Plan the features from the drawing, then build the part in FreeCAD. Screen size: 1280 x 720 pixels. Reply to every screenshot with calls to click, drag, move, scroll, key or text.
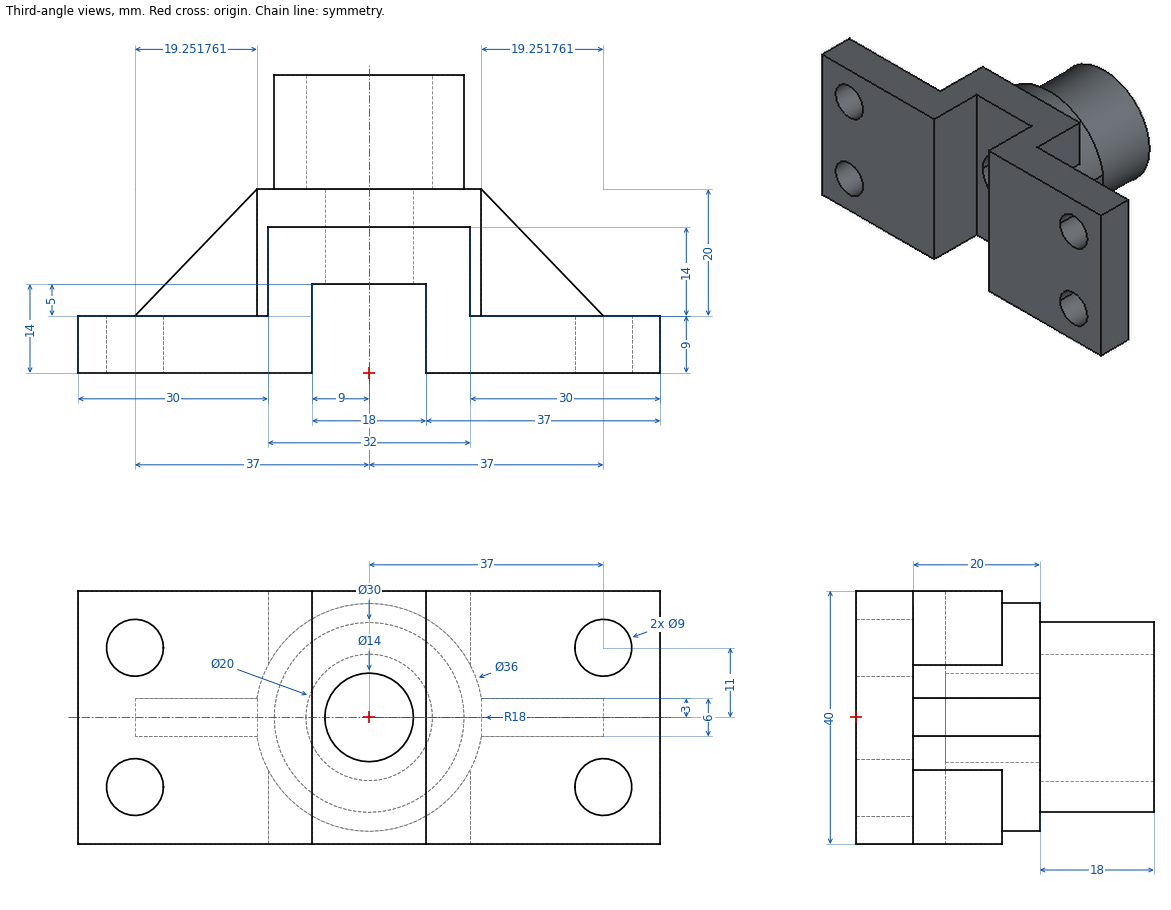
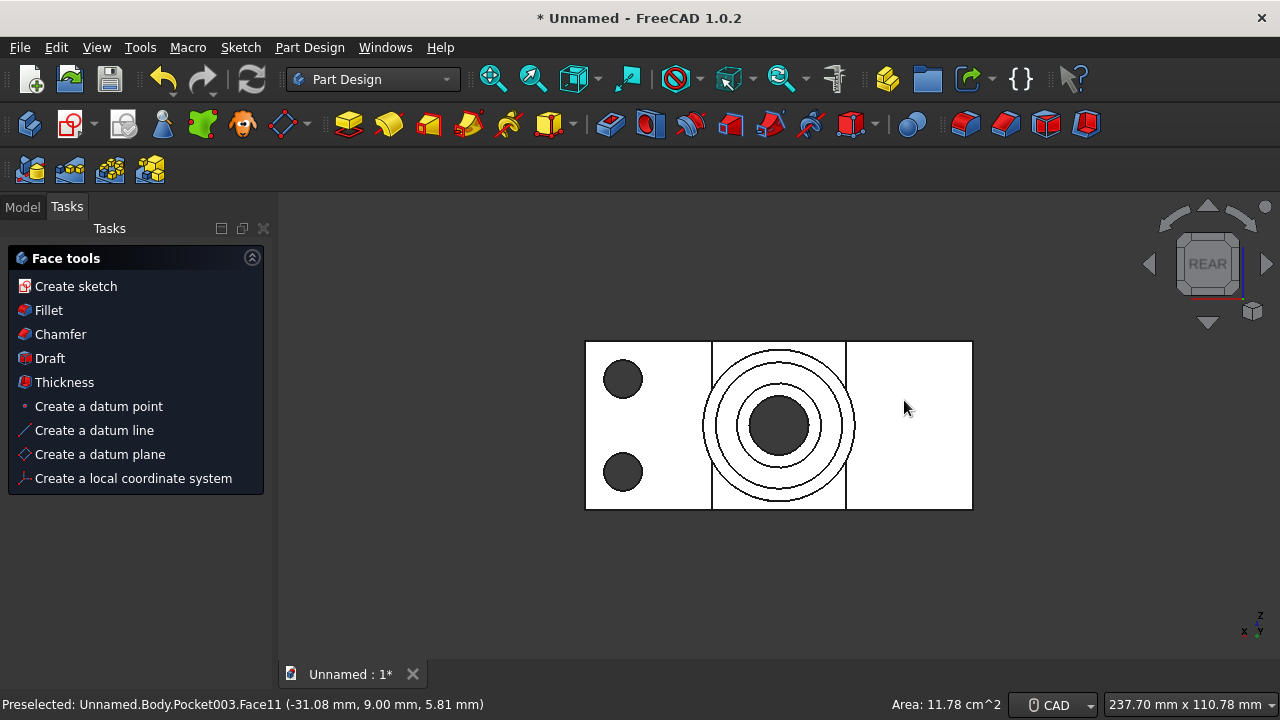
click(70, 124)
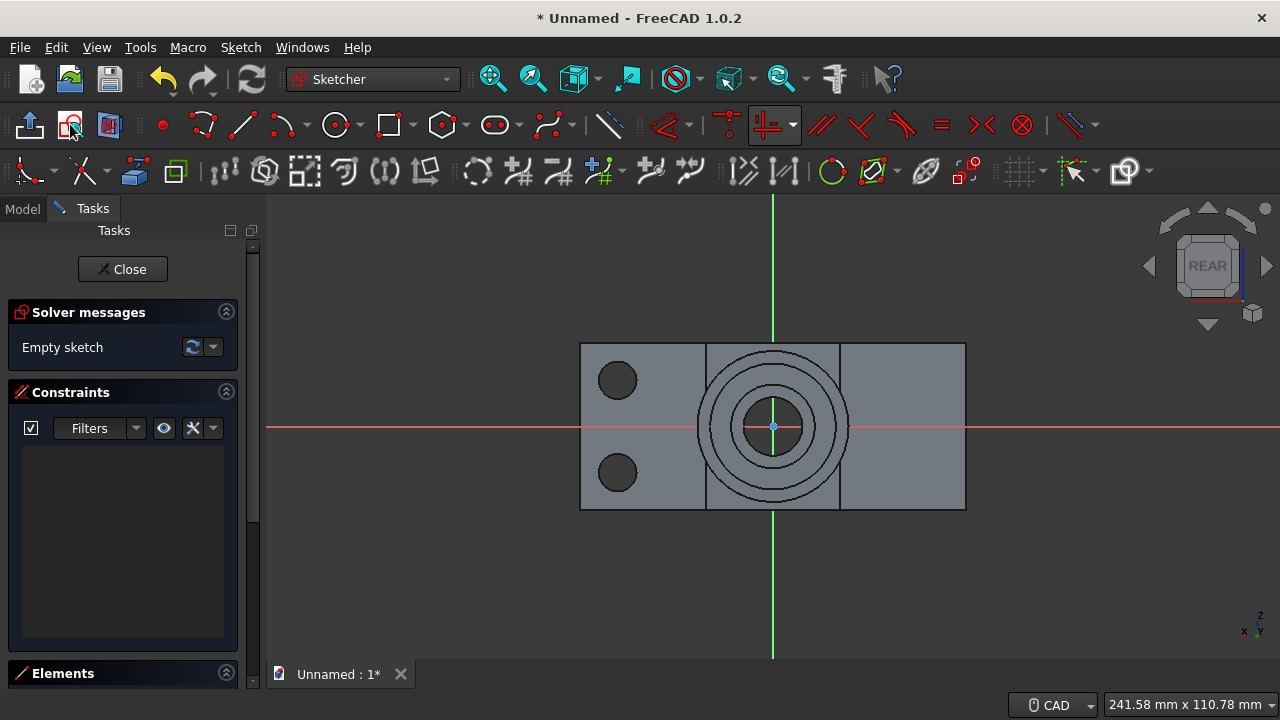
key(q)
key(s)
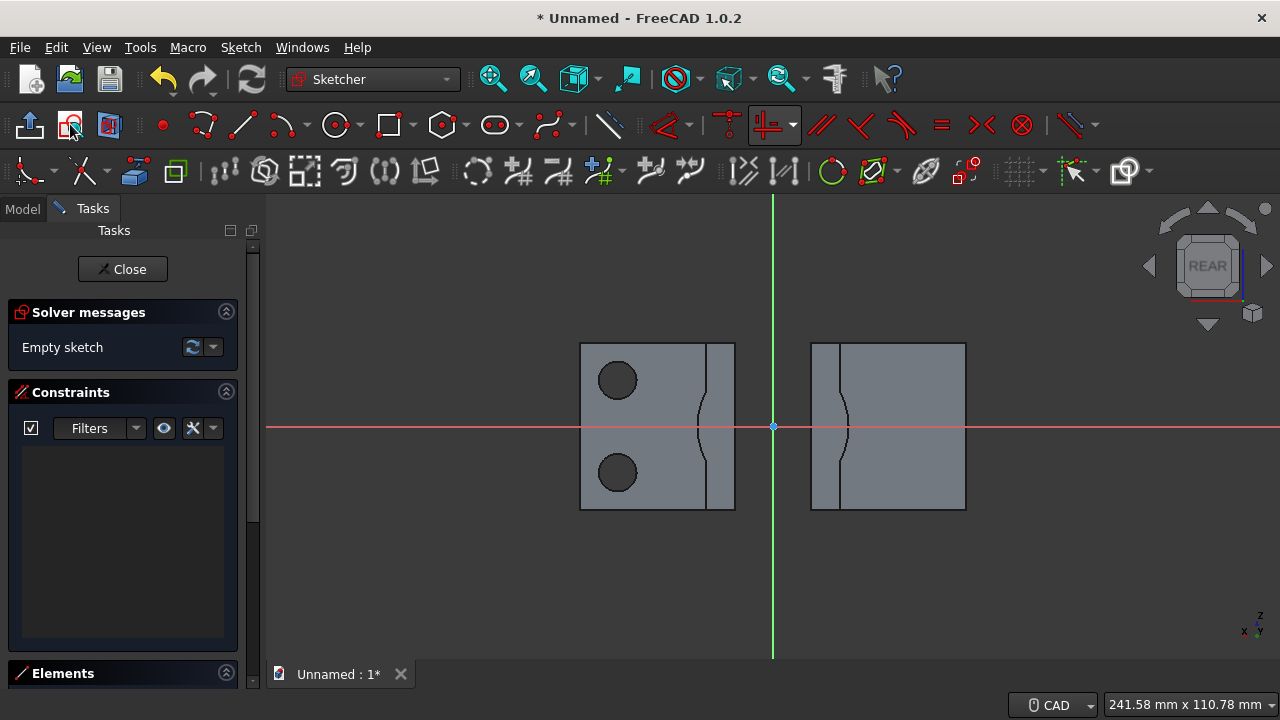
scroll(692, 426, up, 7)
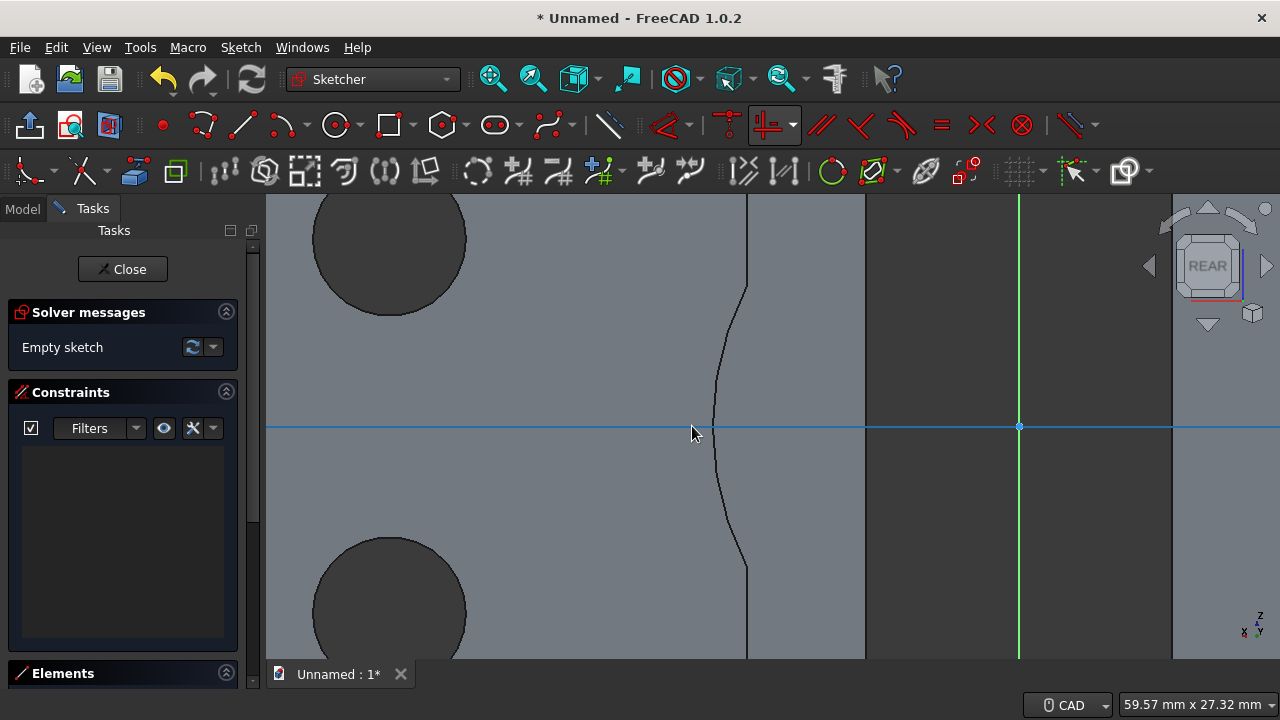
key(g)
key(m)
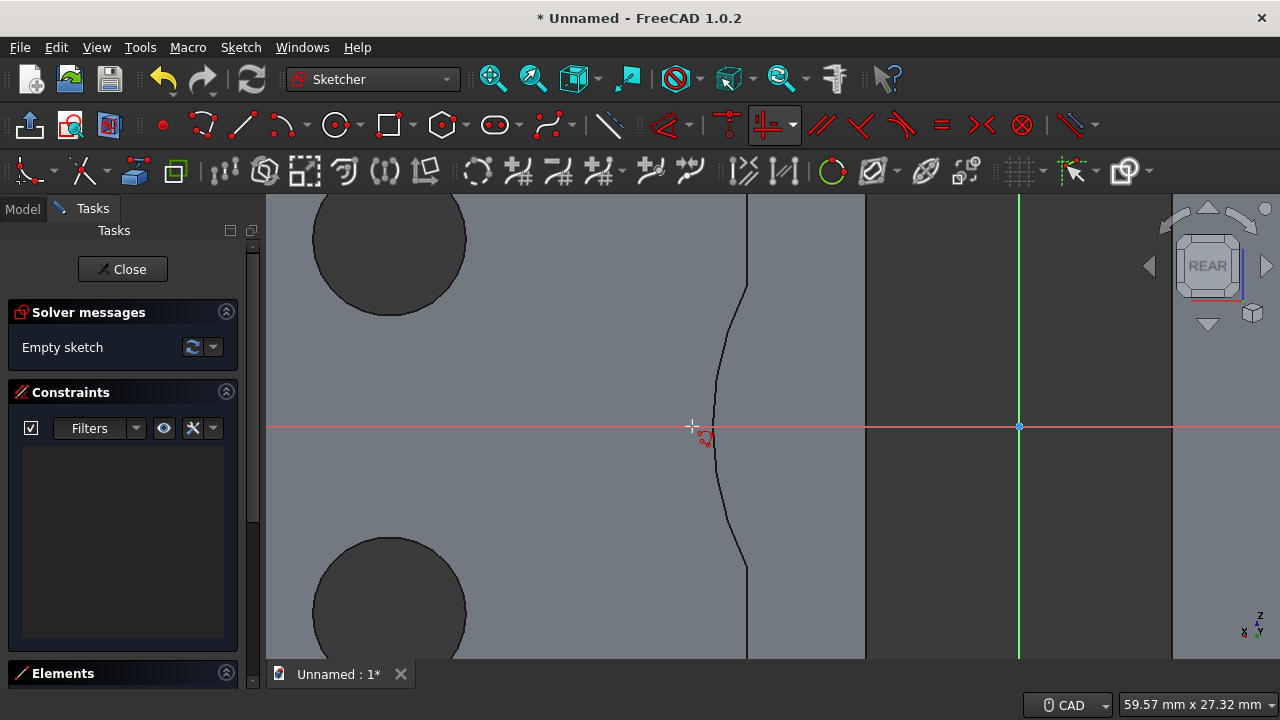
click(717, 375)
click(389, 375)
click(389, 478)
click(717, 478)
right_click(717, 478)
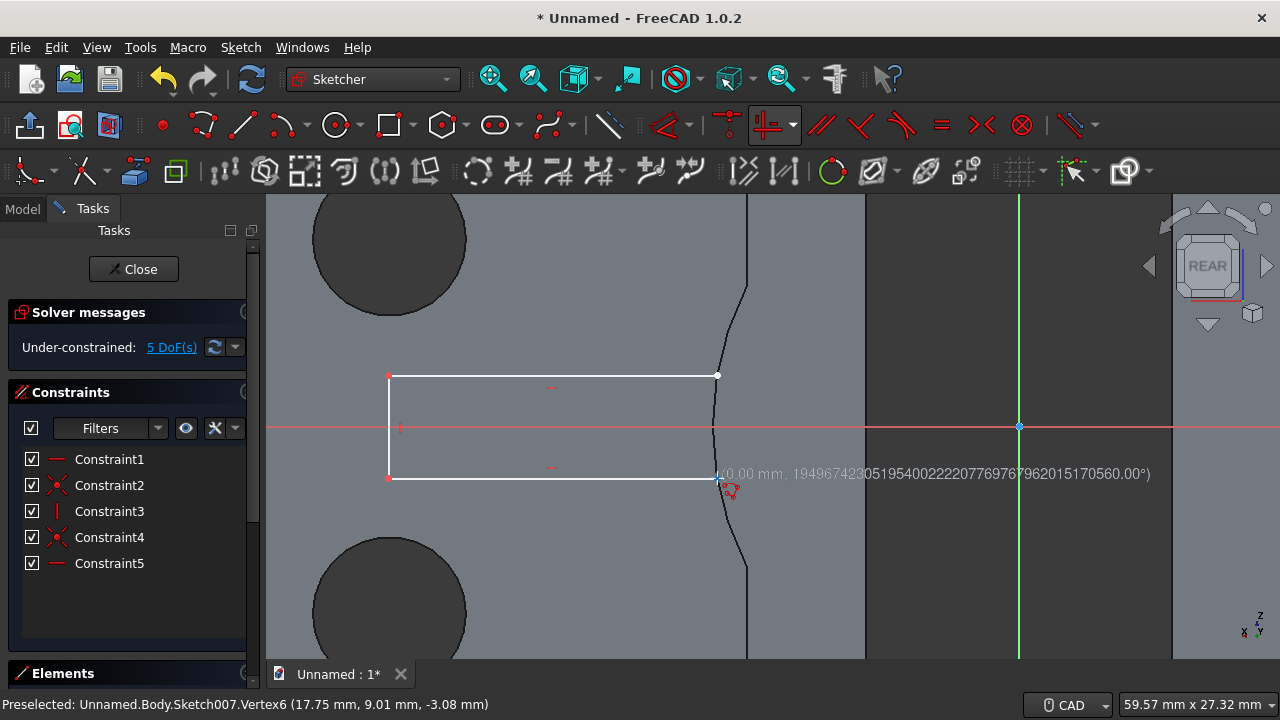
click(310, 126)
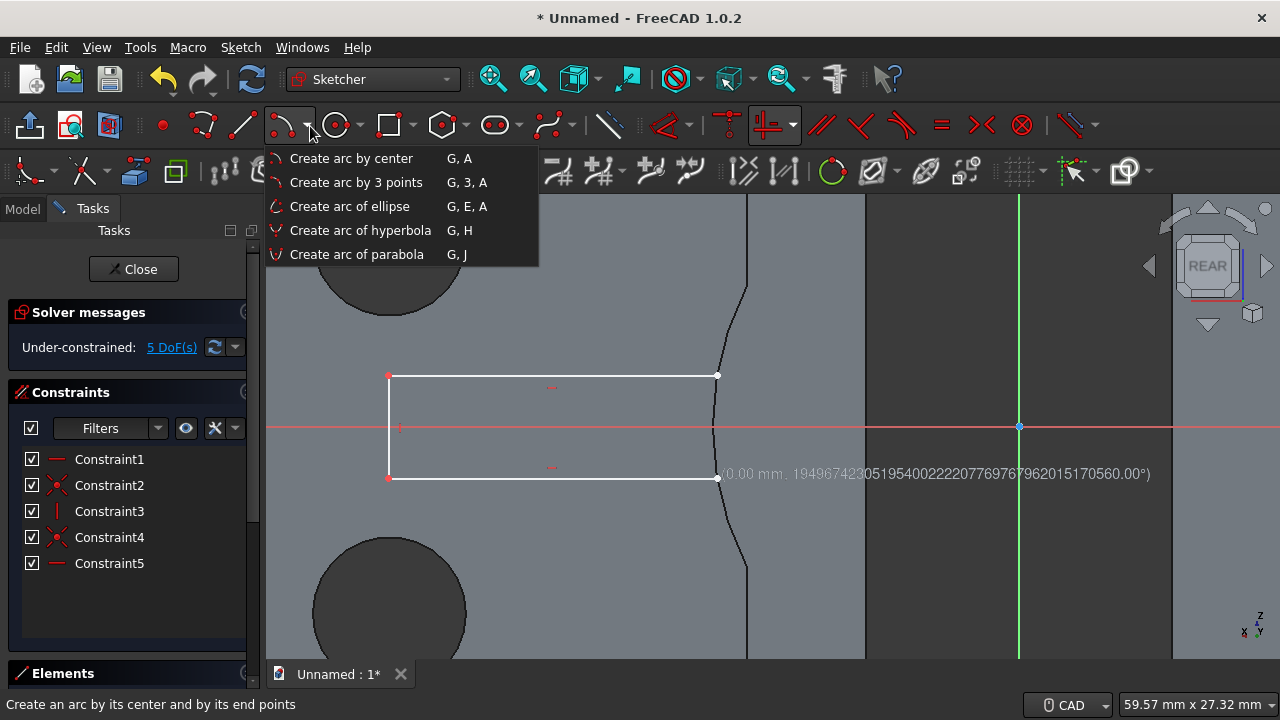
click(402, 182)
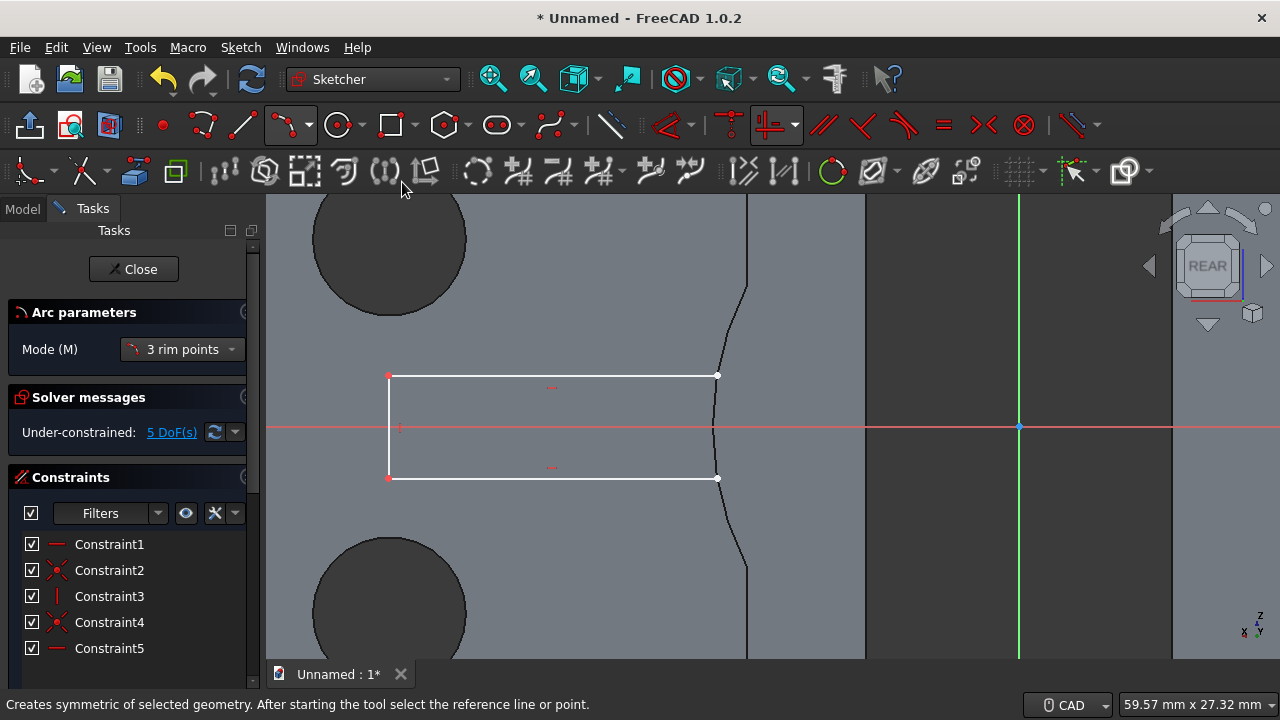
click(717, 479)
click(717, 376)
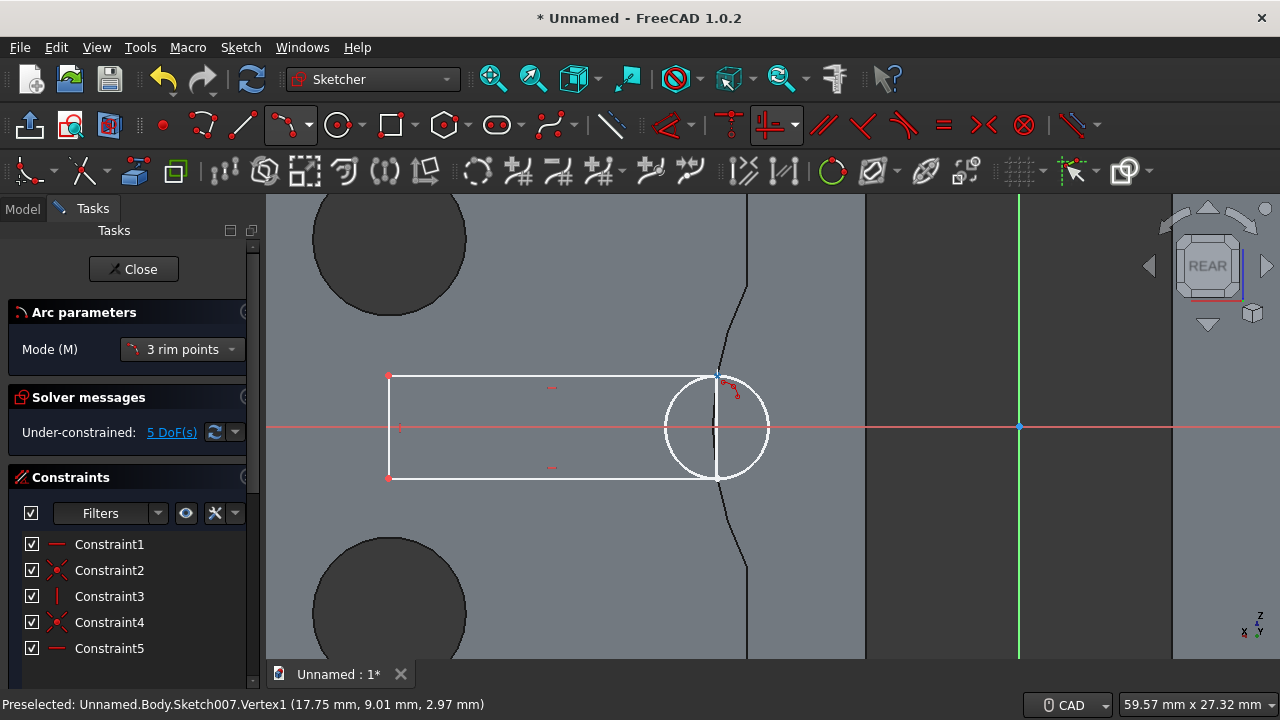
scroll(713, 416, up, 7)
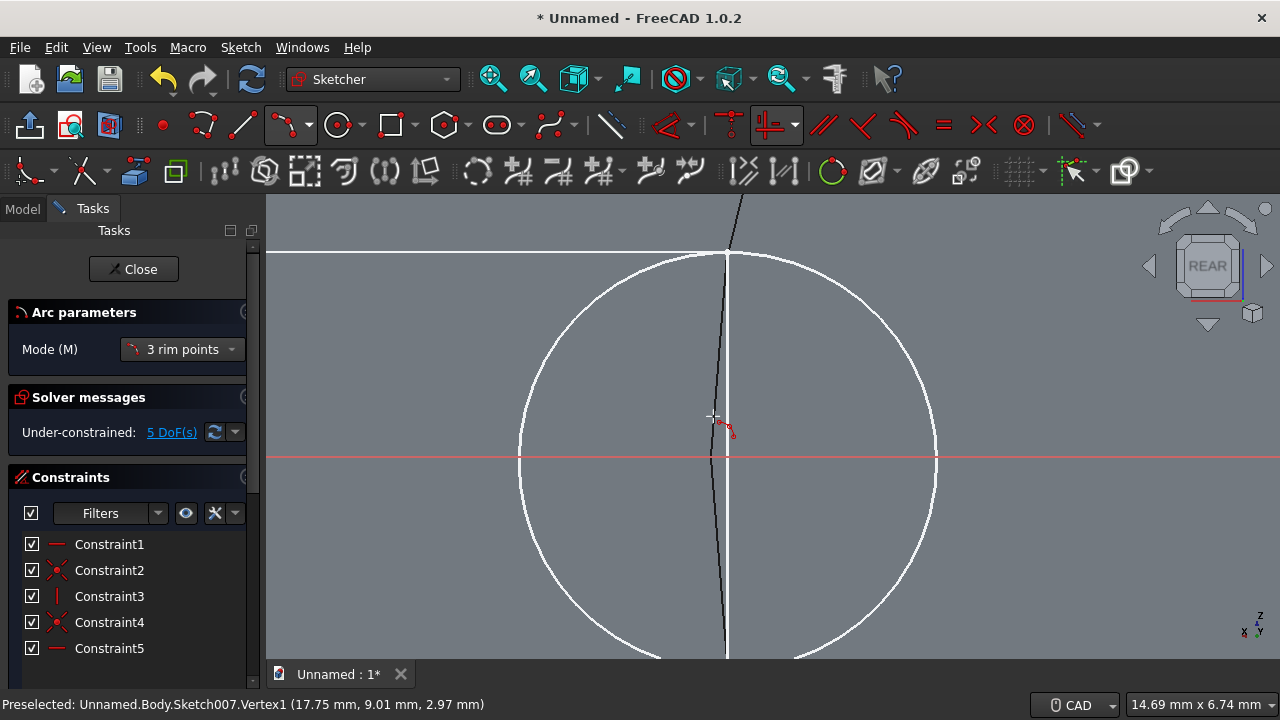
click(712, 416)
key(Escape)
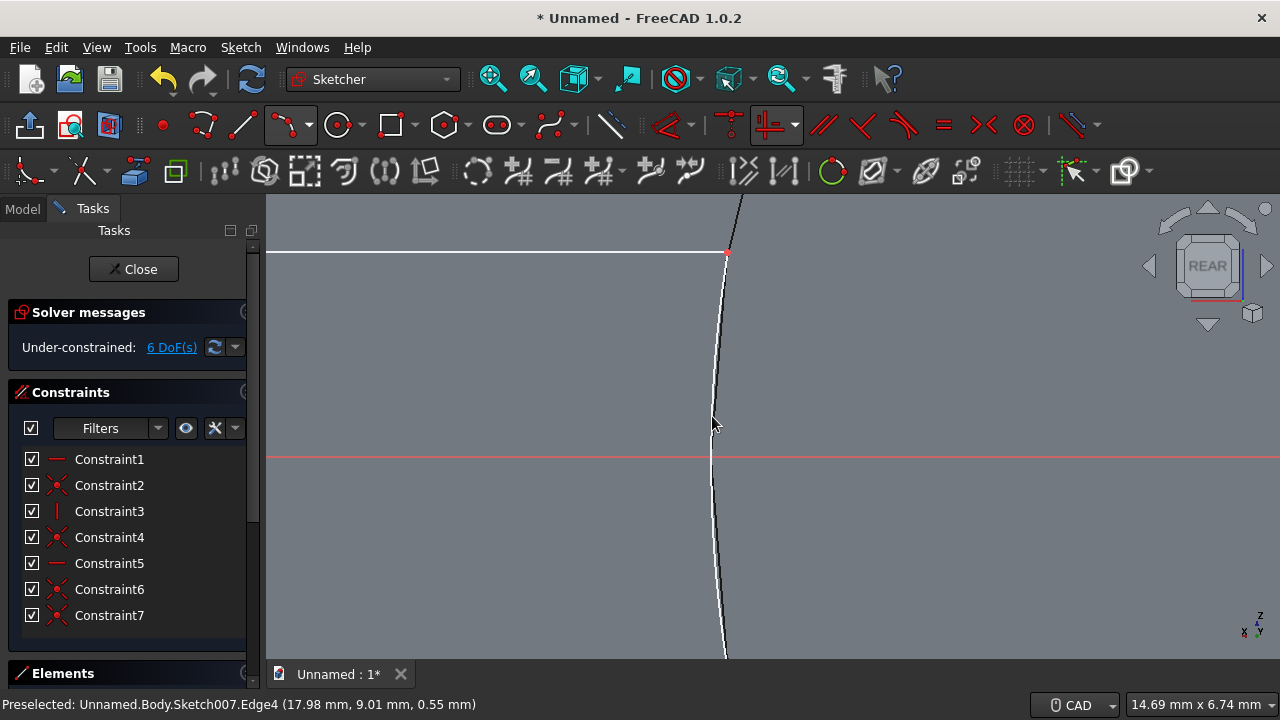
scroll(714, 416, down, 7)